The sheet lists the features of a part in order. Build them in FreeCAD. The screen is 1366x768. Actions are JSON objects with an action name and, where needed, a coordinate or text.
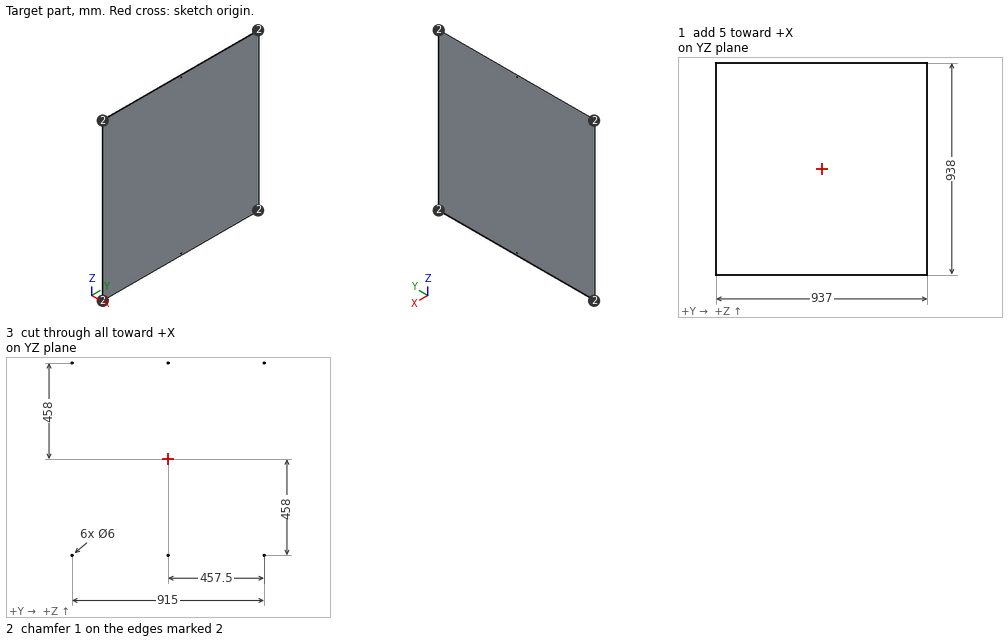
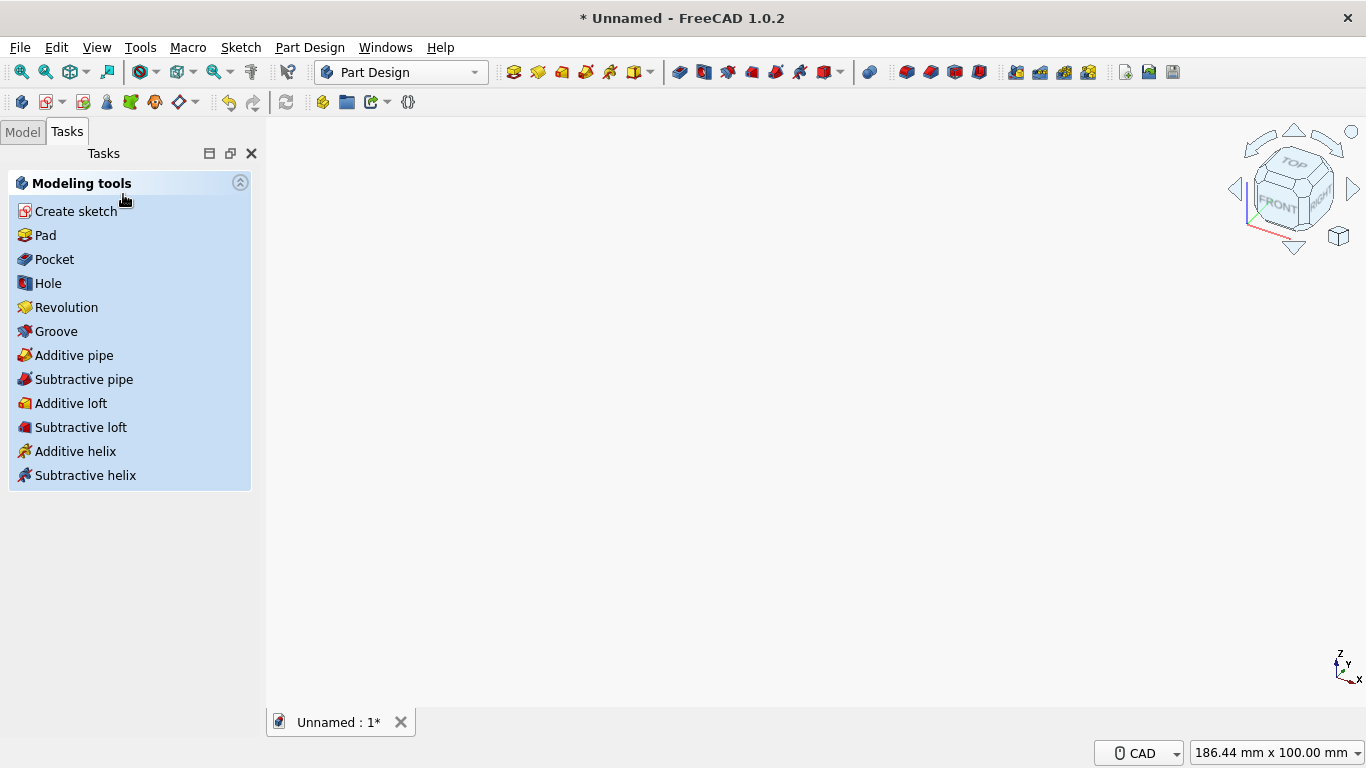
{"action": "left_click", "coordinate": [514, 72]}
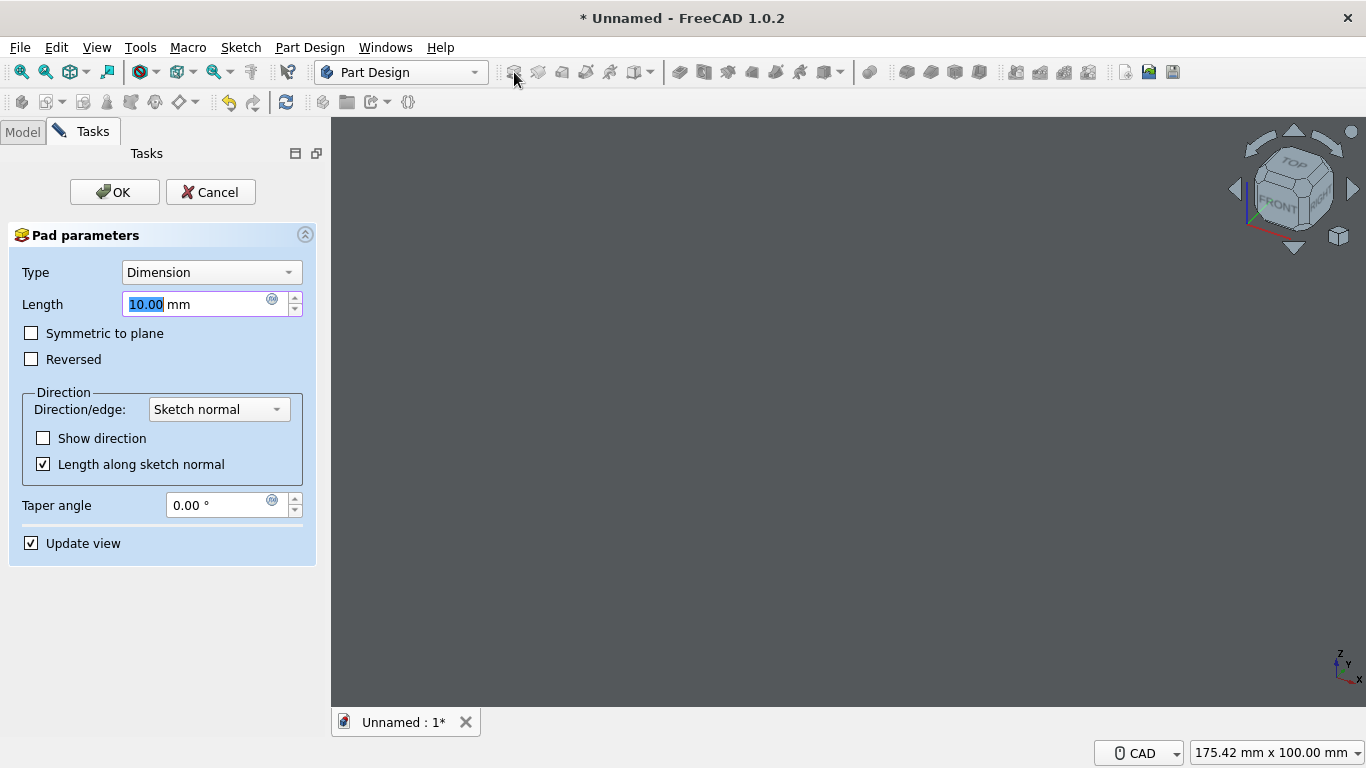
{"action": "type", "text": "5"}
{"action": "key", "text": "Tab"}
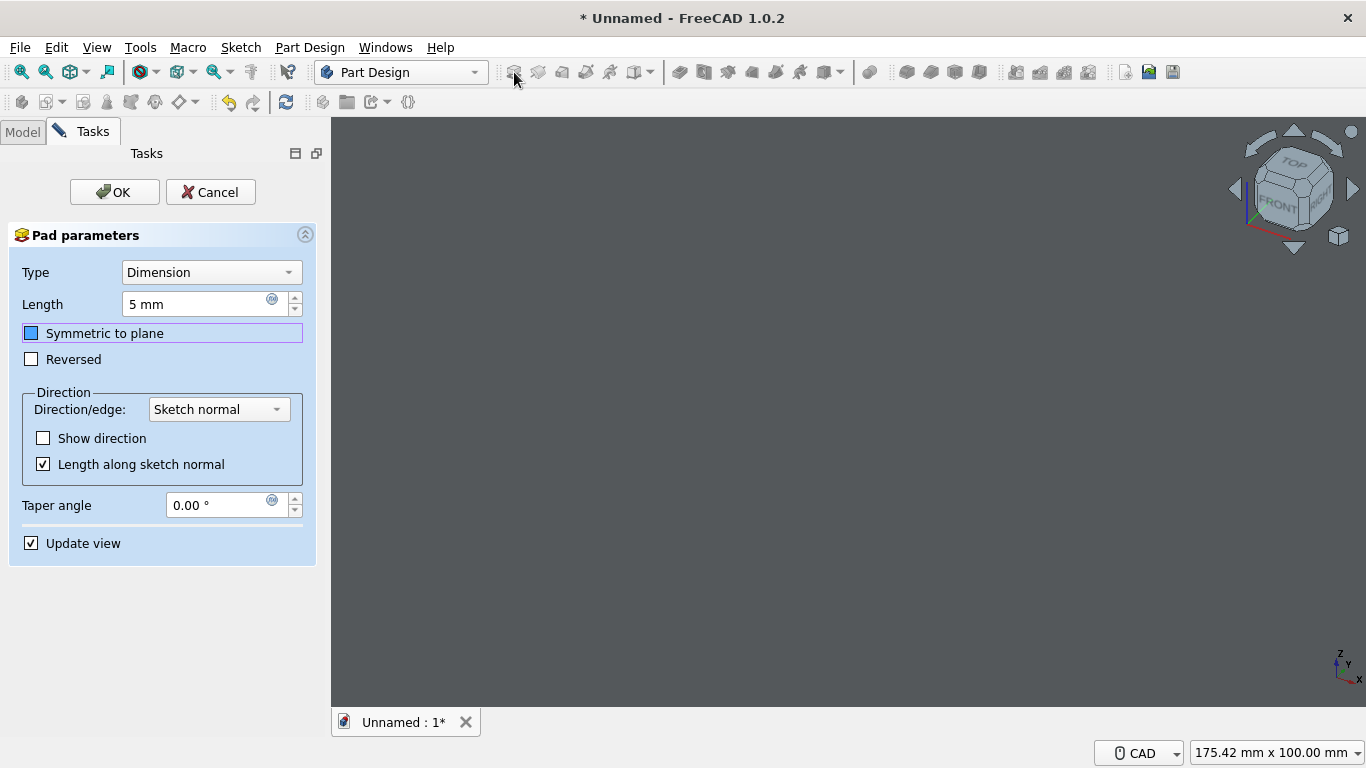
{"action": "left_click", "coordinate": [115, 192]}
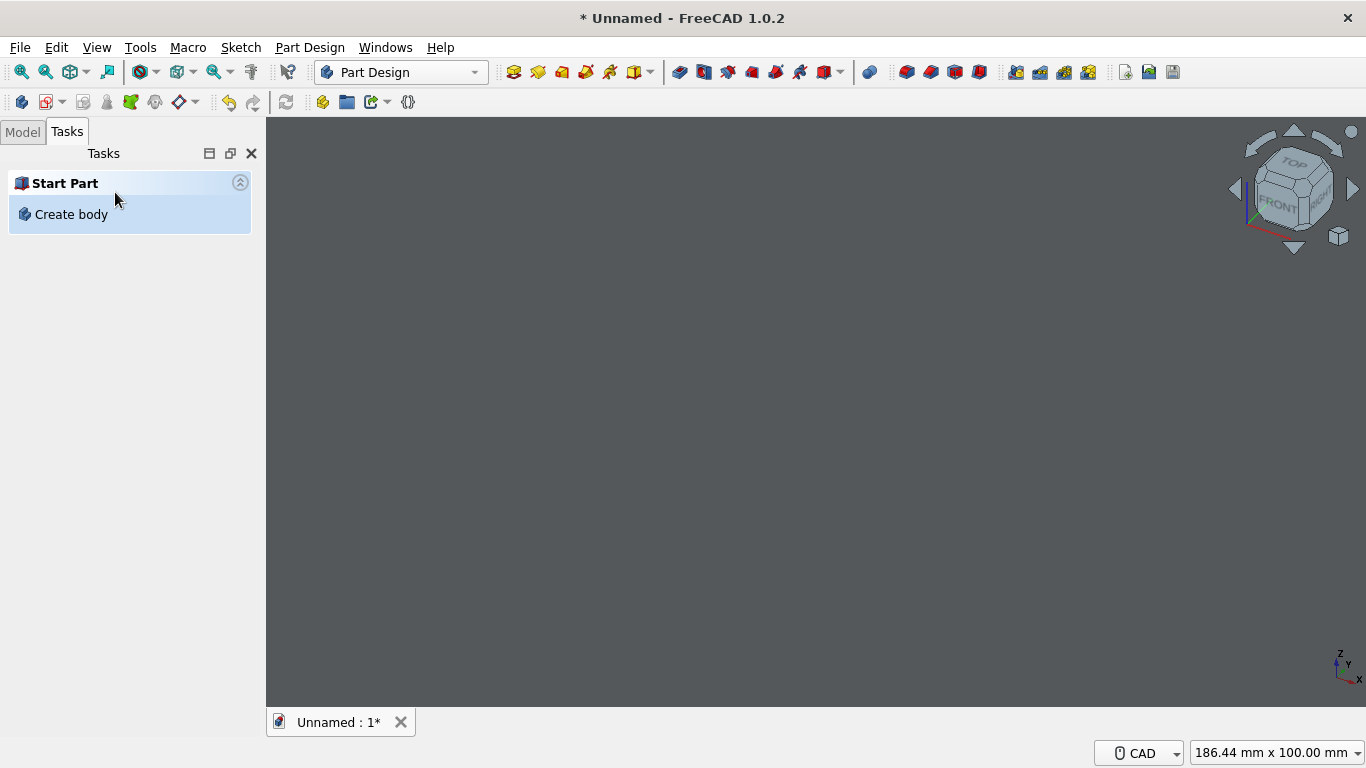
{"action": "left_click", "coordinate": [22, 72]}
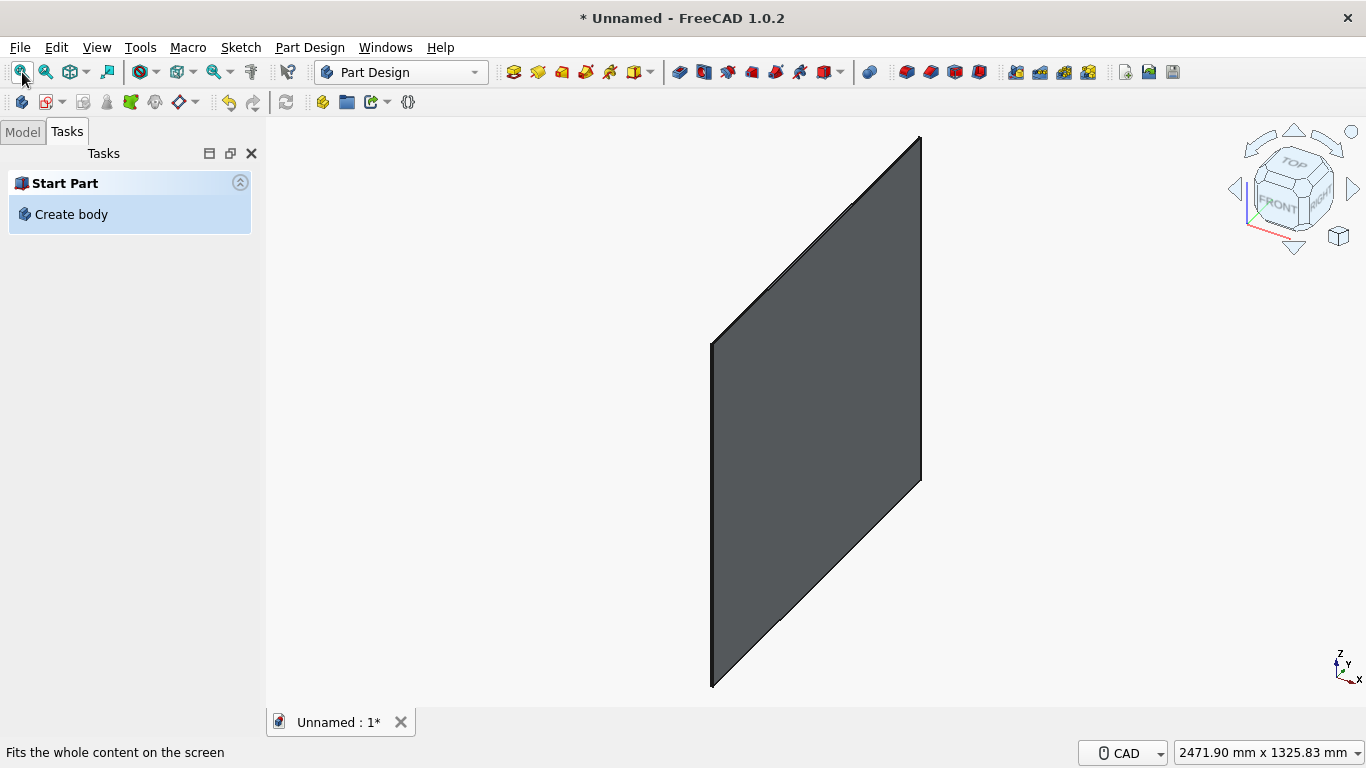
{"action": "key", "text": "0"}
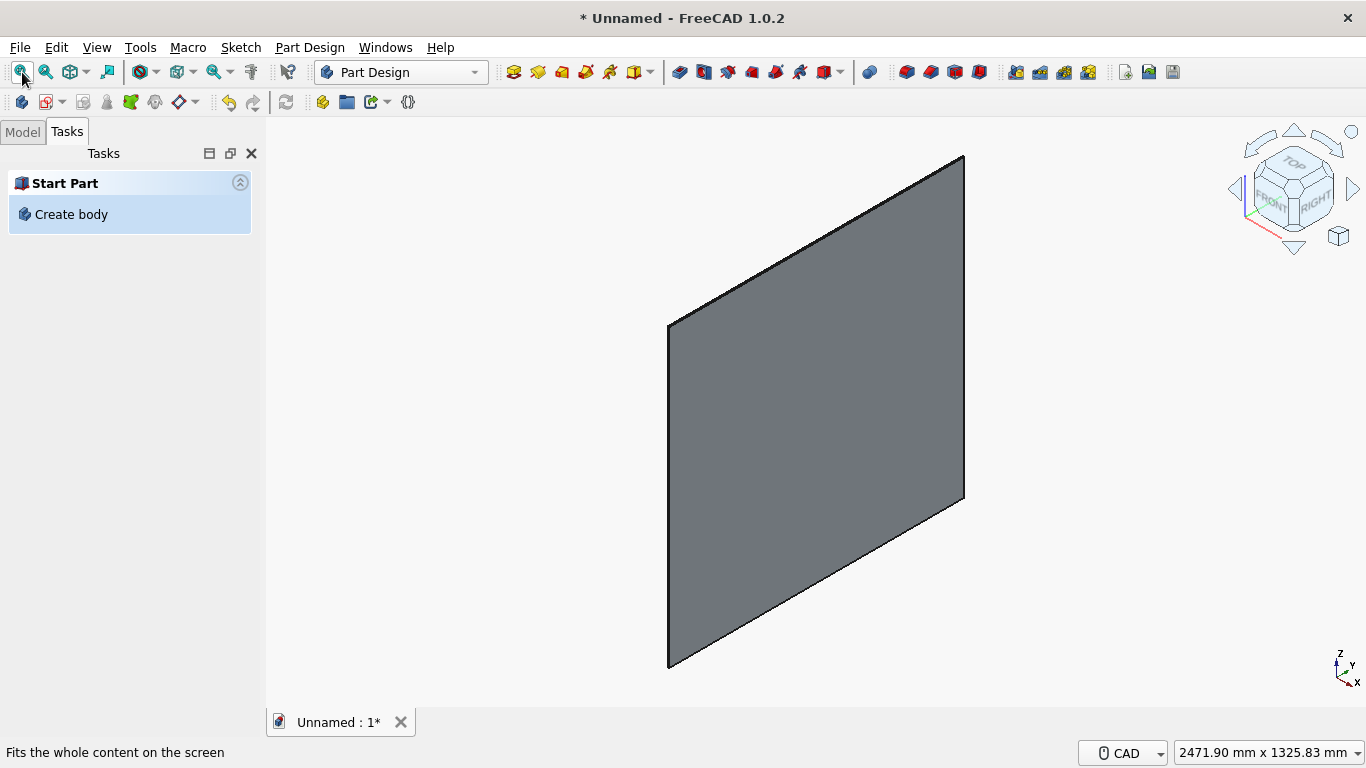
{"action": "scroll", "coordinate": [963, 155], "scroll_direction": "up", "scroll_amount": 15}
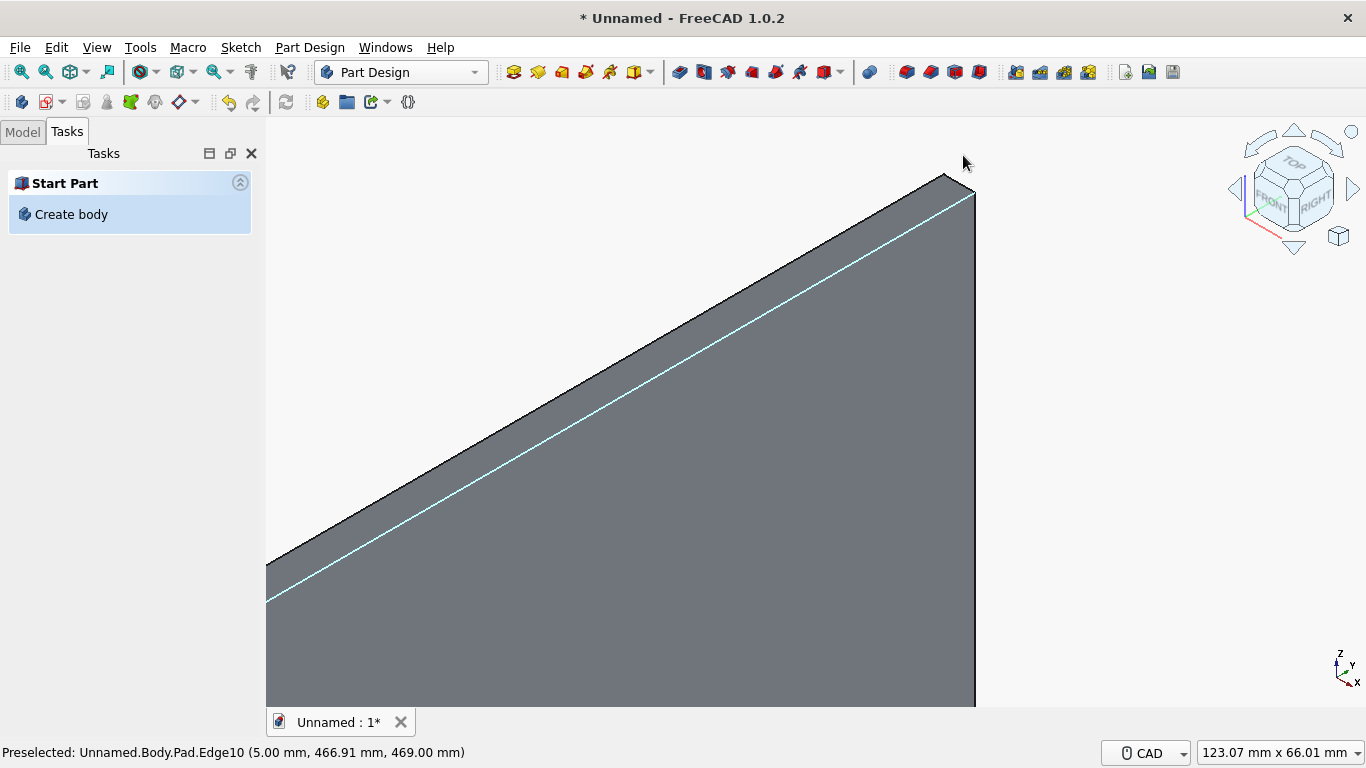
{"action": "left_click", "coordinate": [22, 72]}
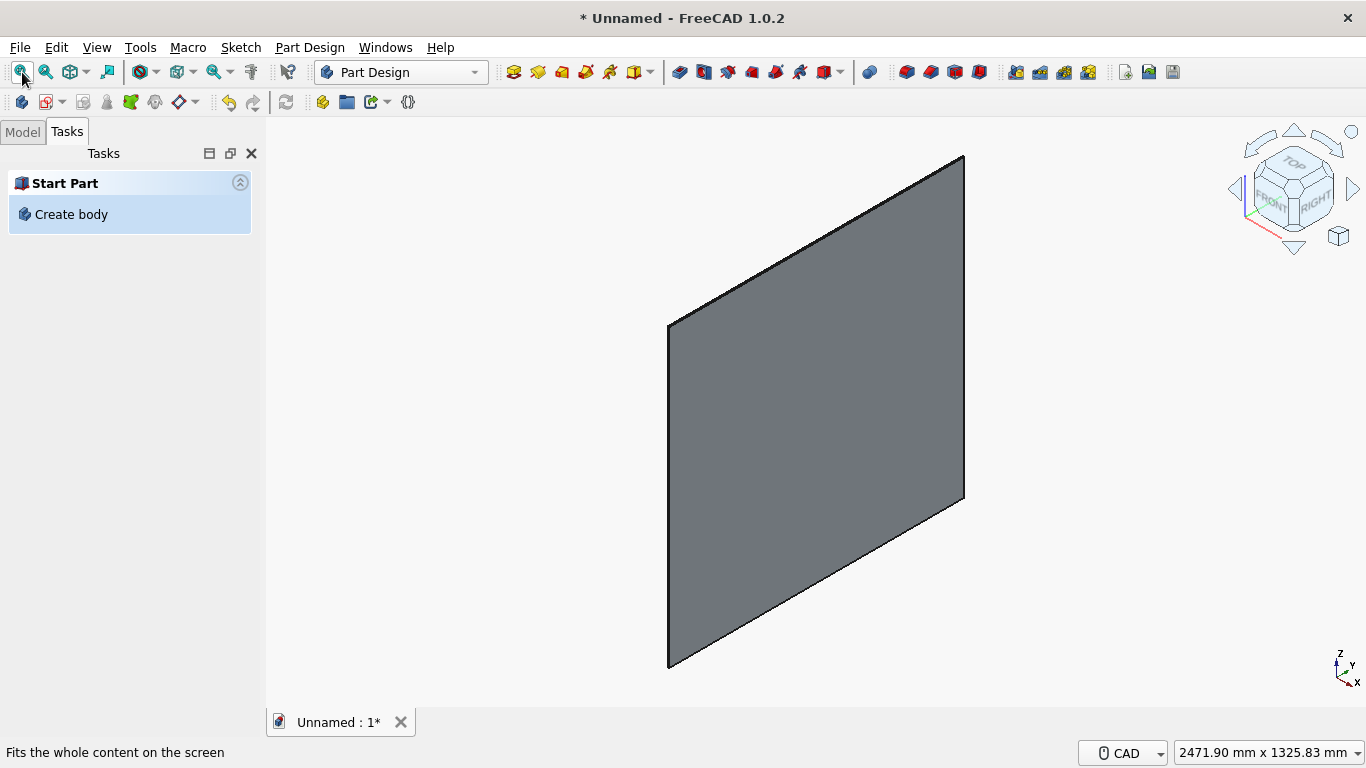
{"action": "key", "text": "2"}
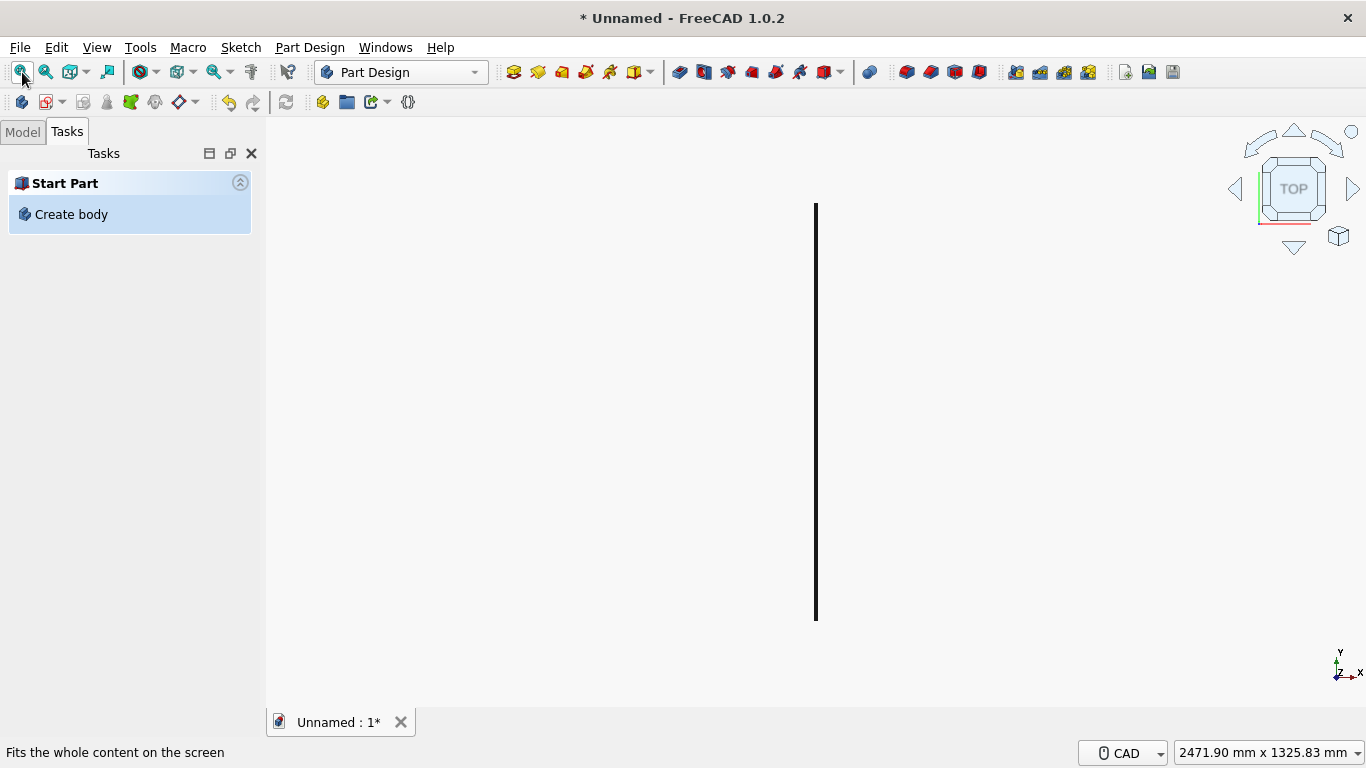
{"action": "scroll", "coordinate": [816, 203], "scroll_direction": "up", "scroll_amount": 15}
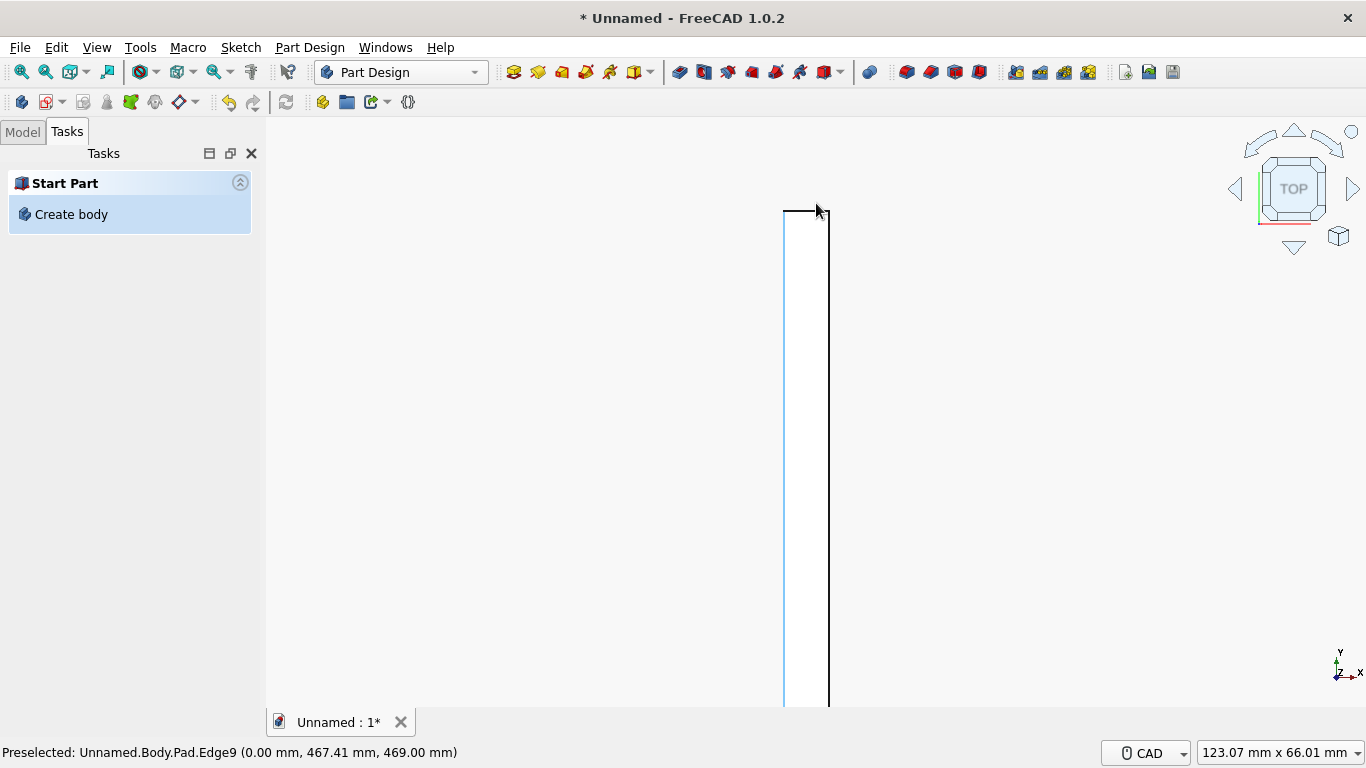
{"action": "left_click", "coordinate": [806, 210]}